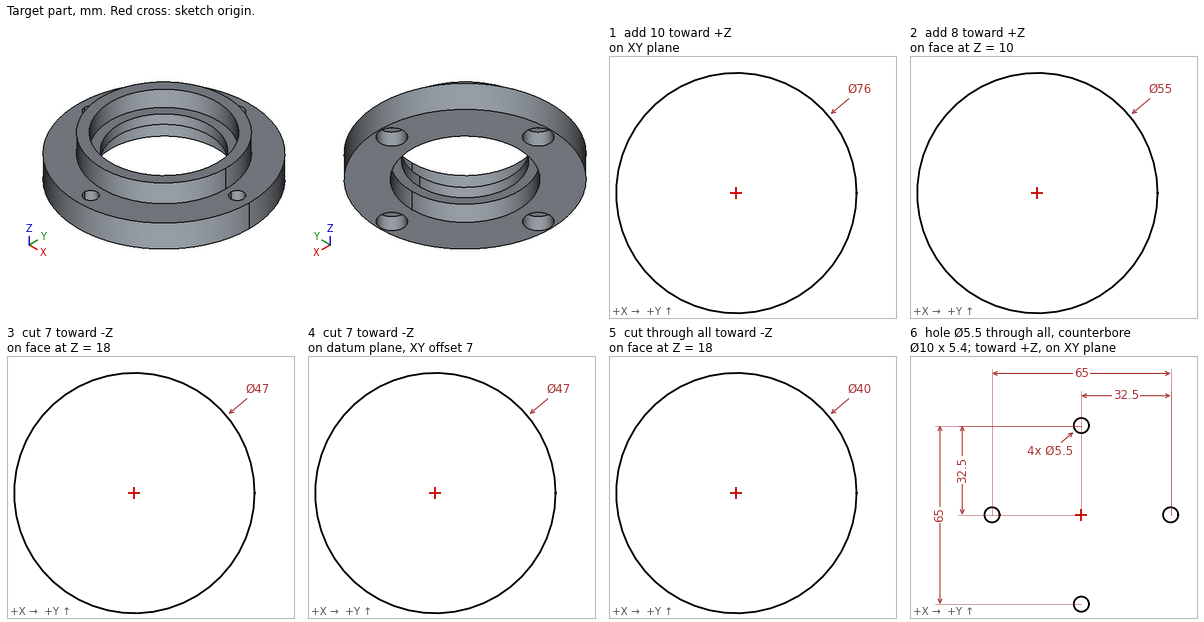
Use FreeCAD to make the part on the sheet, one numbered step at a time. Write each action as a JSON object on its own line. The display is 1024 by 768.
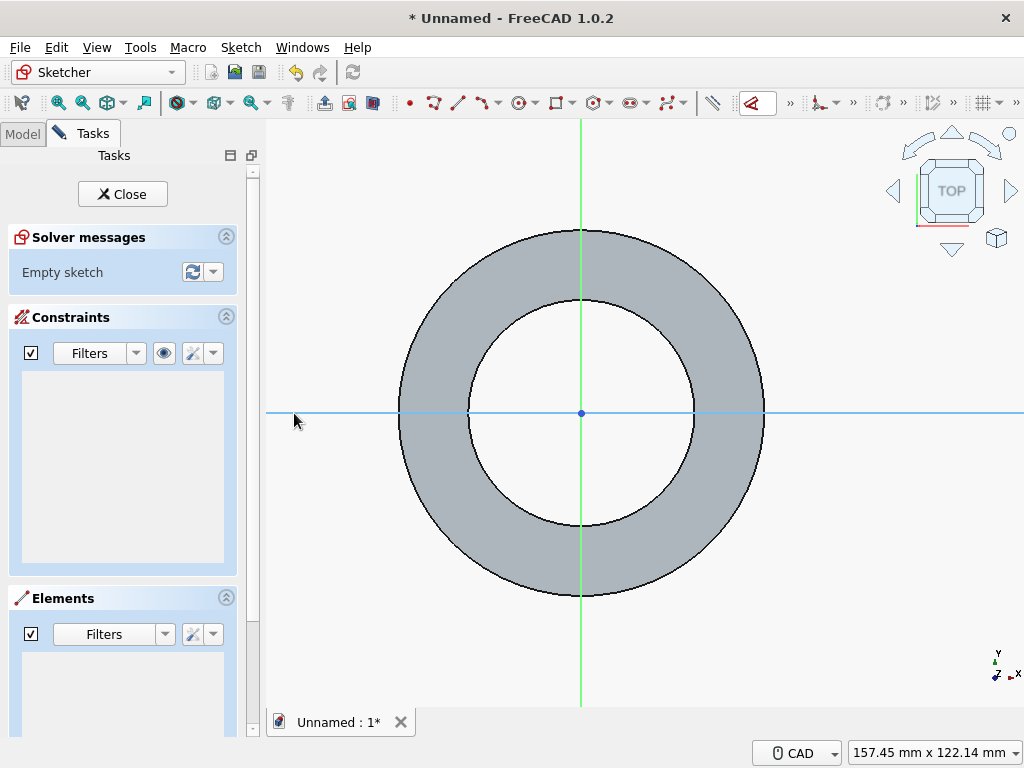
{"action": "key", "text": "g c"}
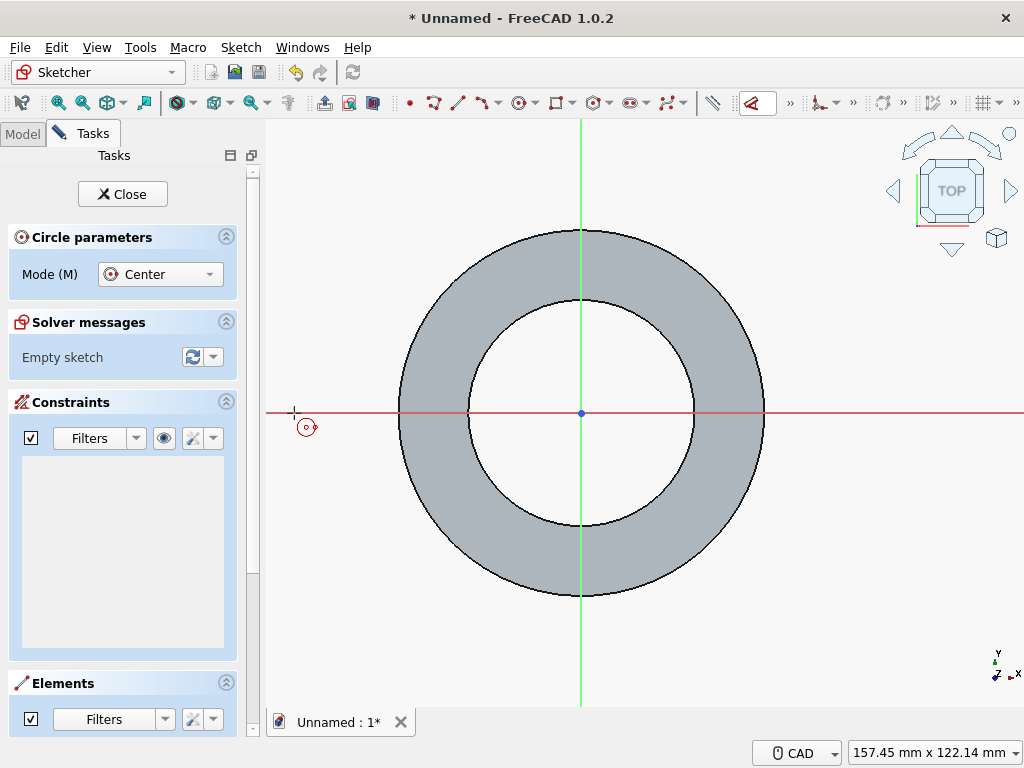
{"action": "scroll", "coordinate": [581, 257], "scroll_direction": "up", "scroll_amount": 3}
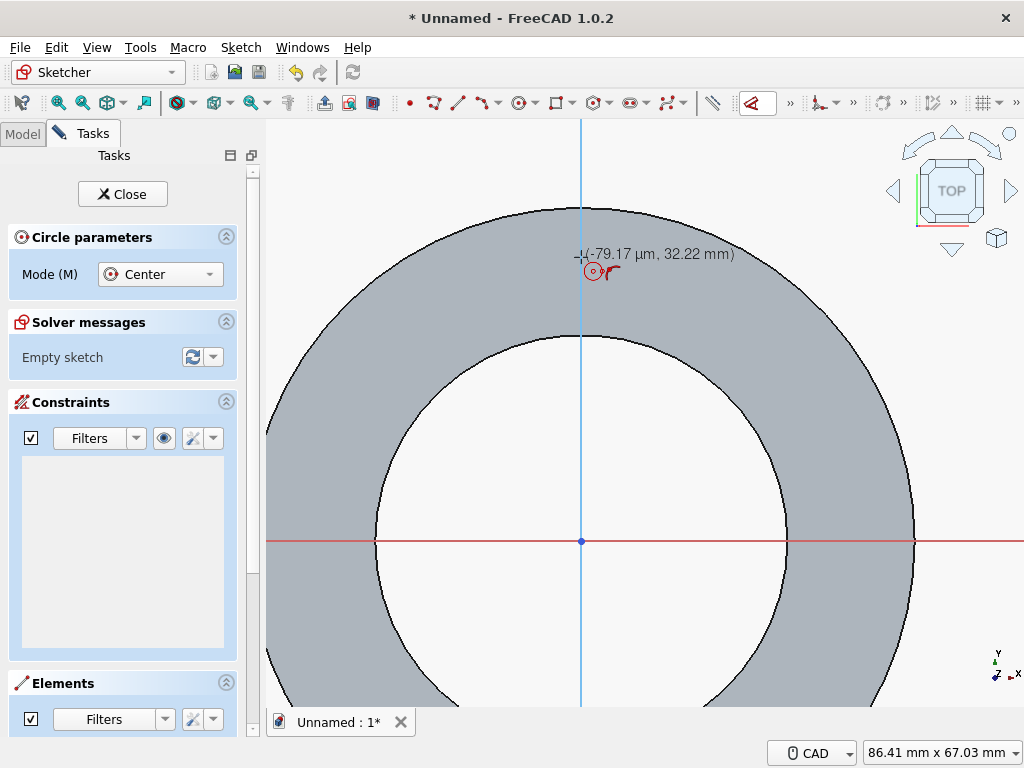
{"action": "left_click", "coordinate": [581, 256]}
{"action": "left_click", "coordinate": [598, 239]}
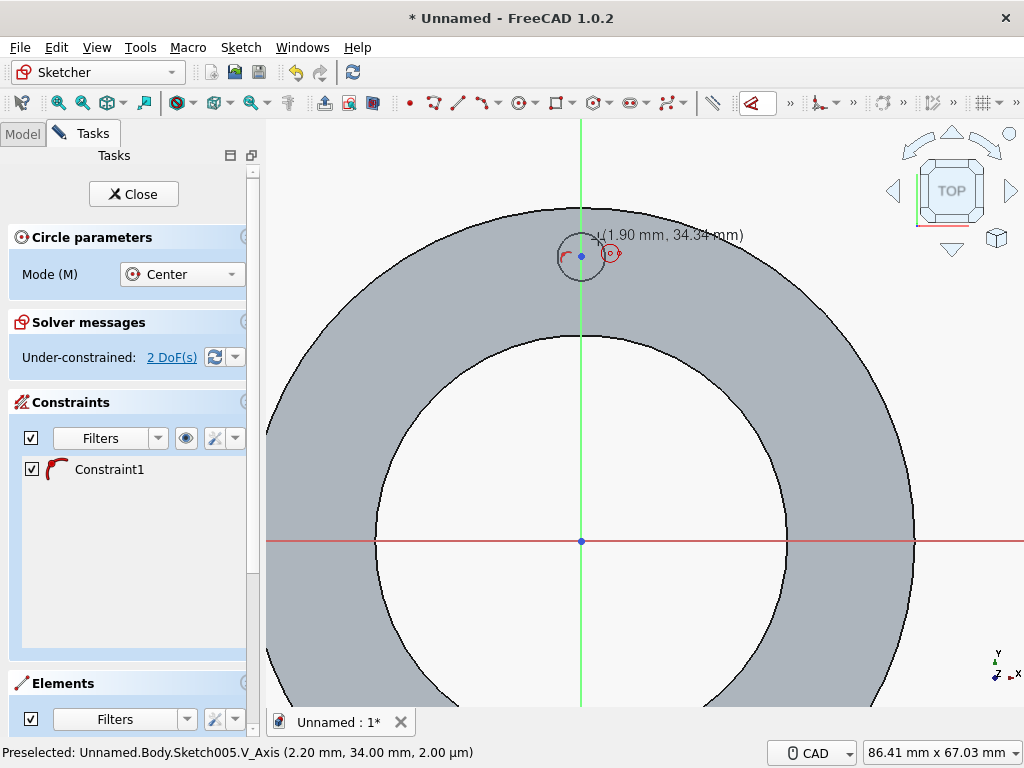
{"action": "scroll", "coordinate": [567, 152], "scroll_direction": "down", "scroll_amount": 2}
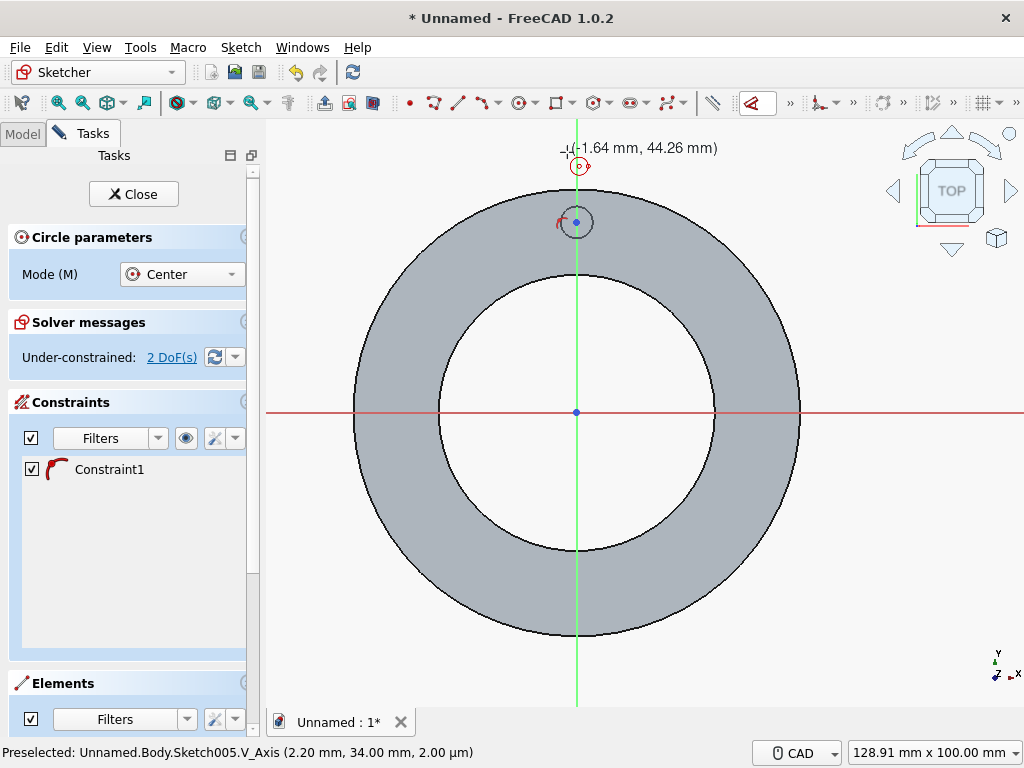
{"action": "scroll", "coordinate": [768, 413], "scroll_direction": "up", "scroll_amount": 2}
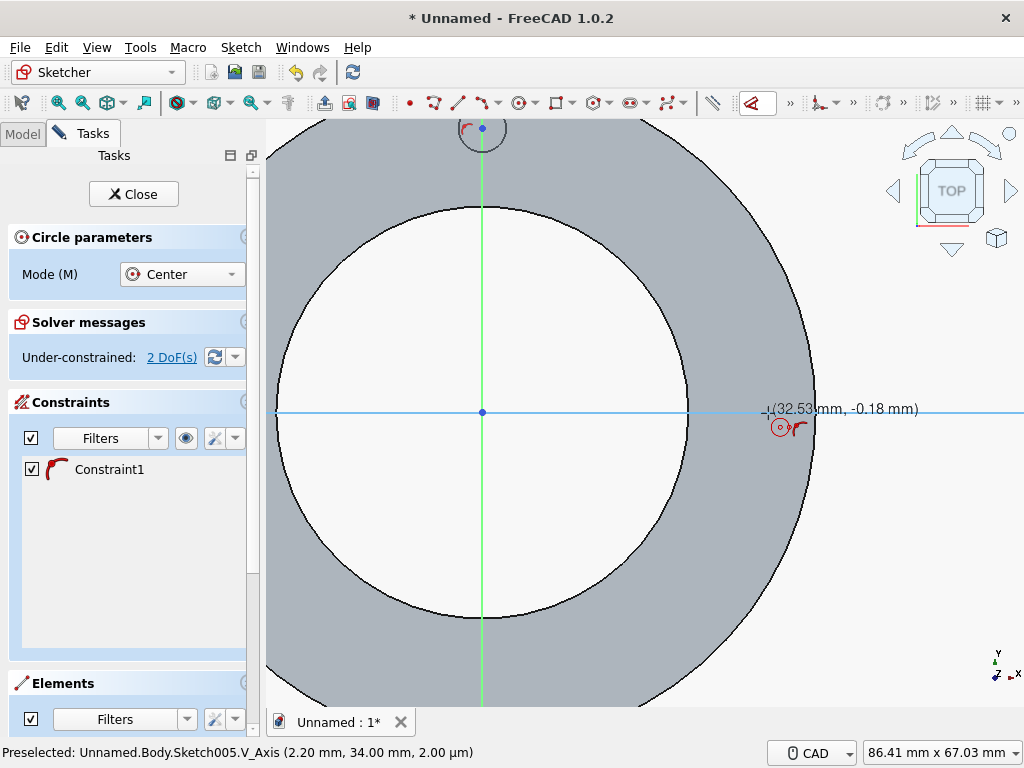
{"action": "left_click", "coordinate": [767, 413]}
{"action": "left_click", "coordinate": [785, 396]}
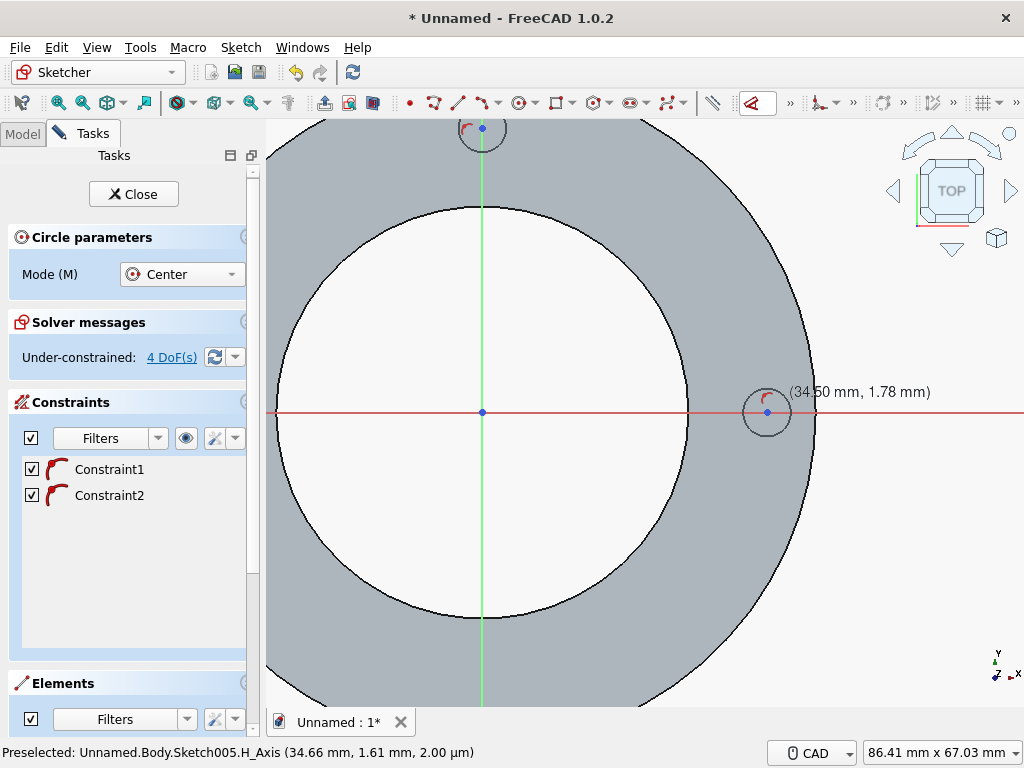
{"action": "scroll", "coordinate": [768, 414], "scroll_direction": "down", "scroll_amount": 2}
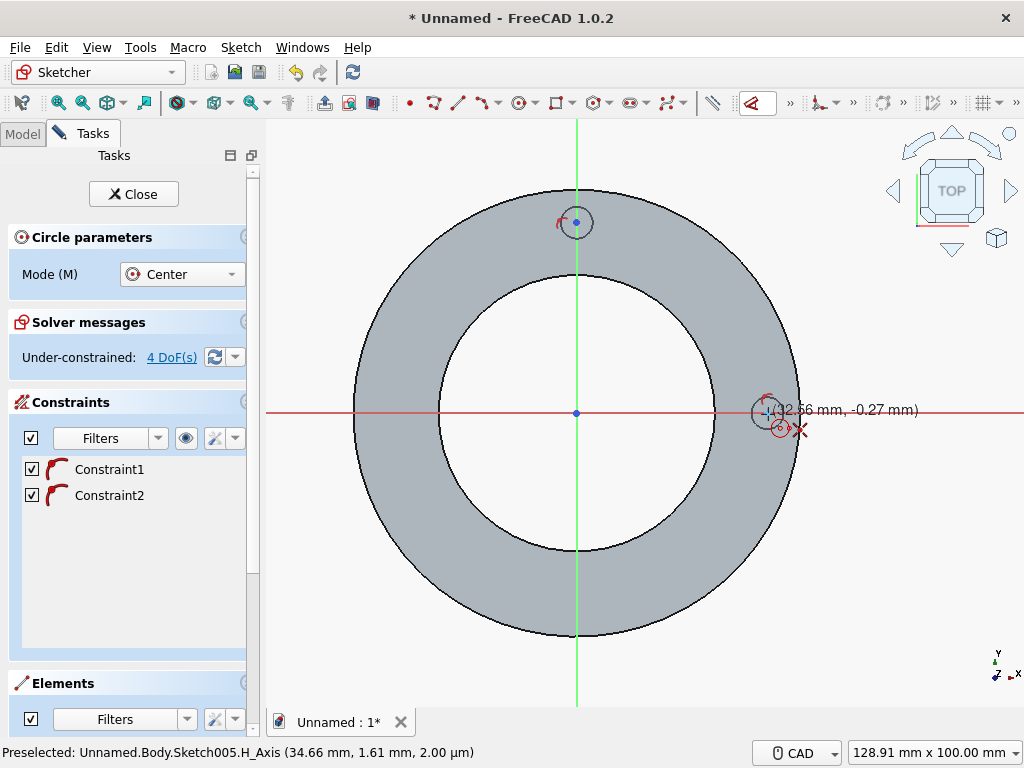
{"action": "scroll", "coordinate": [577, 604], "scroll_direction": "up", "scroll_amount": 2}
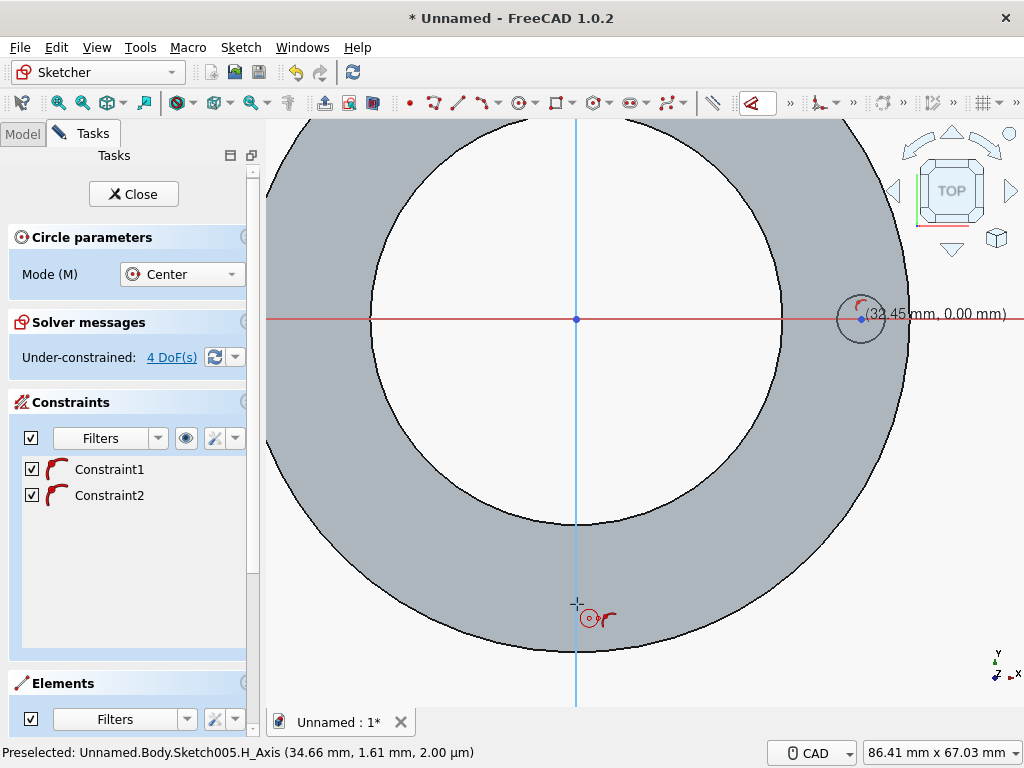
{"action": "left_click", "coordinate": [576, 604]}
{"action": "left_click", "coordinate": [593, 587]}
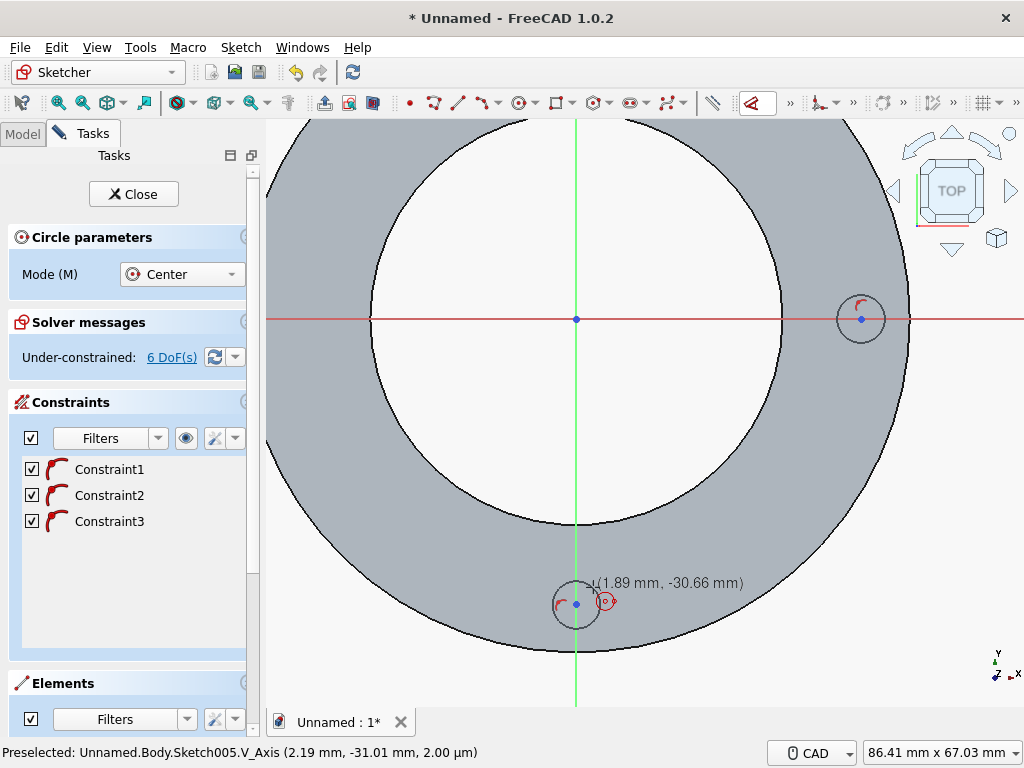
{"action": "scroll", "coordinate": [577, 604], "scroll_direction": "down", "scroll_amount": 2}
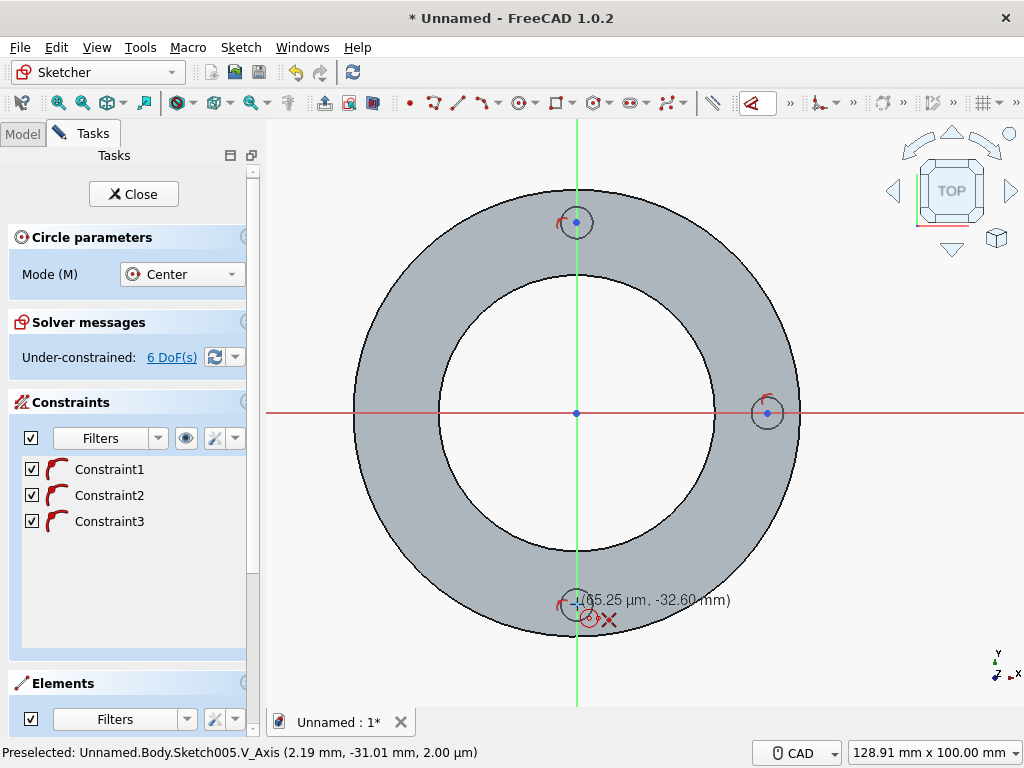
{"action": "scroll", "coordinate": [386, 413], "scroll_direction": "up", "scroll_amount": 2}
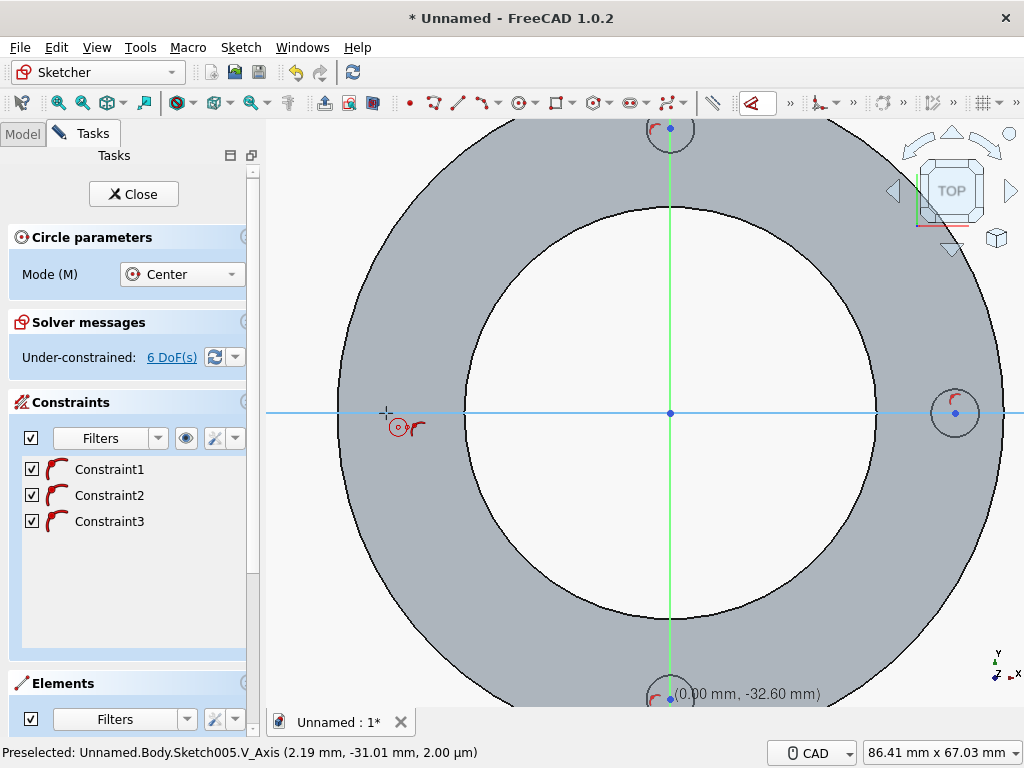
{"action": "left_click", "coordinate": [385, 413]}
{"action": "left_click", "coordinate": [402, 396]}
{"action": "key", "text": "Escape"}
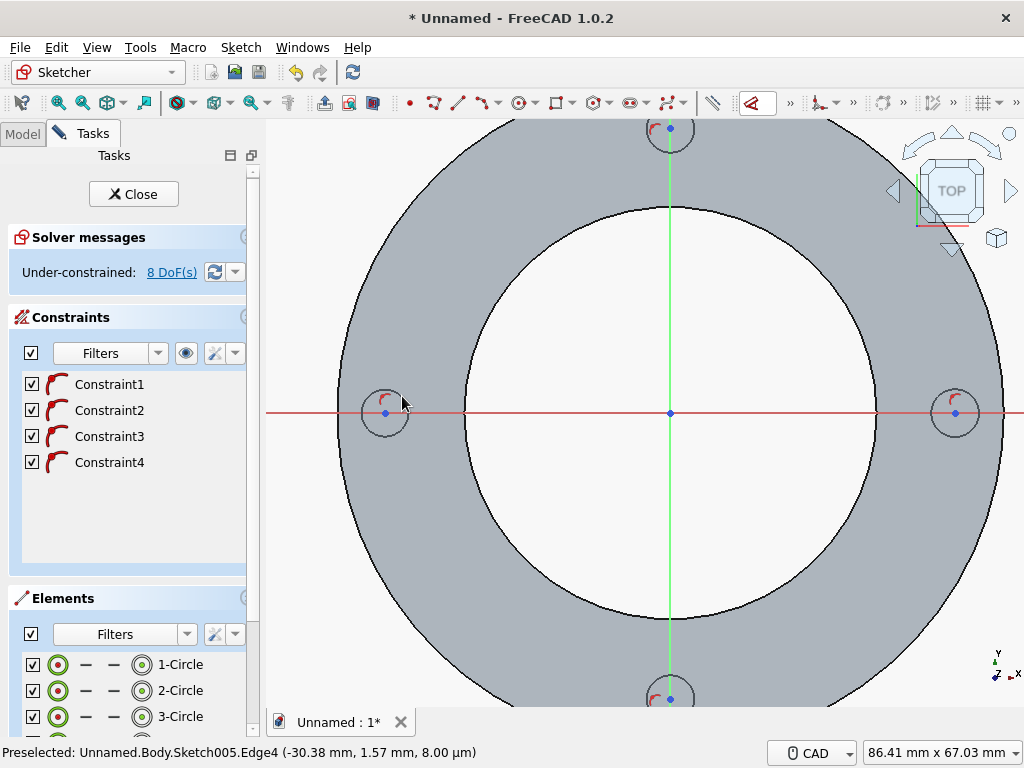
{"action": "left_click", "coordinate": [670, 153]}